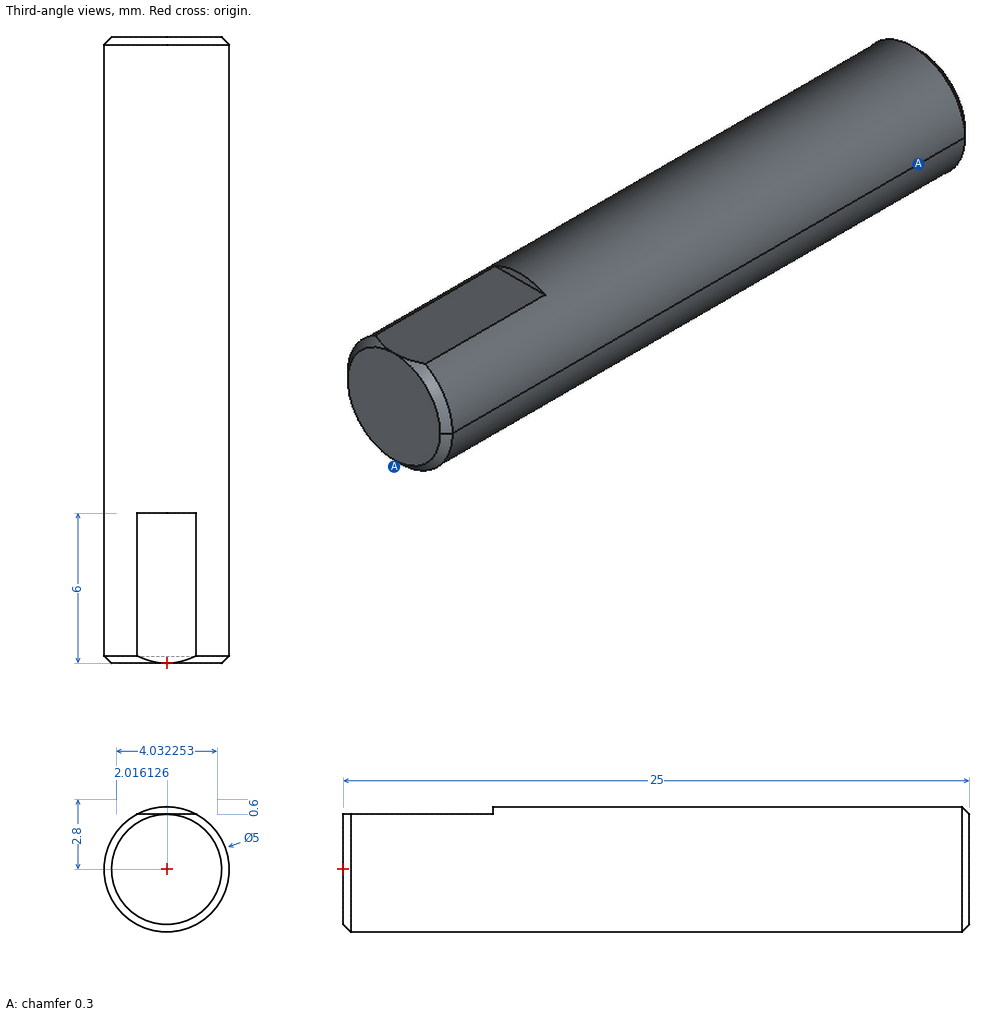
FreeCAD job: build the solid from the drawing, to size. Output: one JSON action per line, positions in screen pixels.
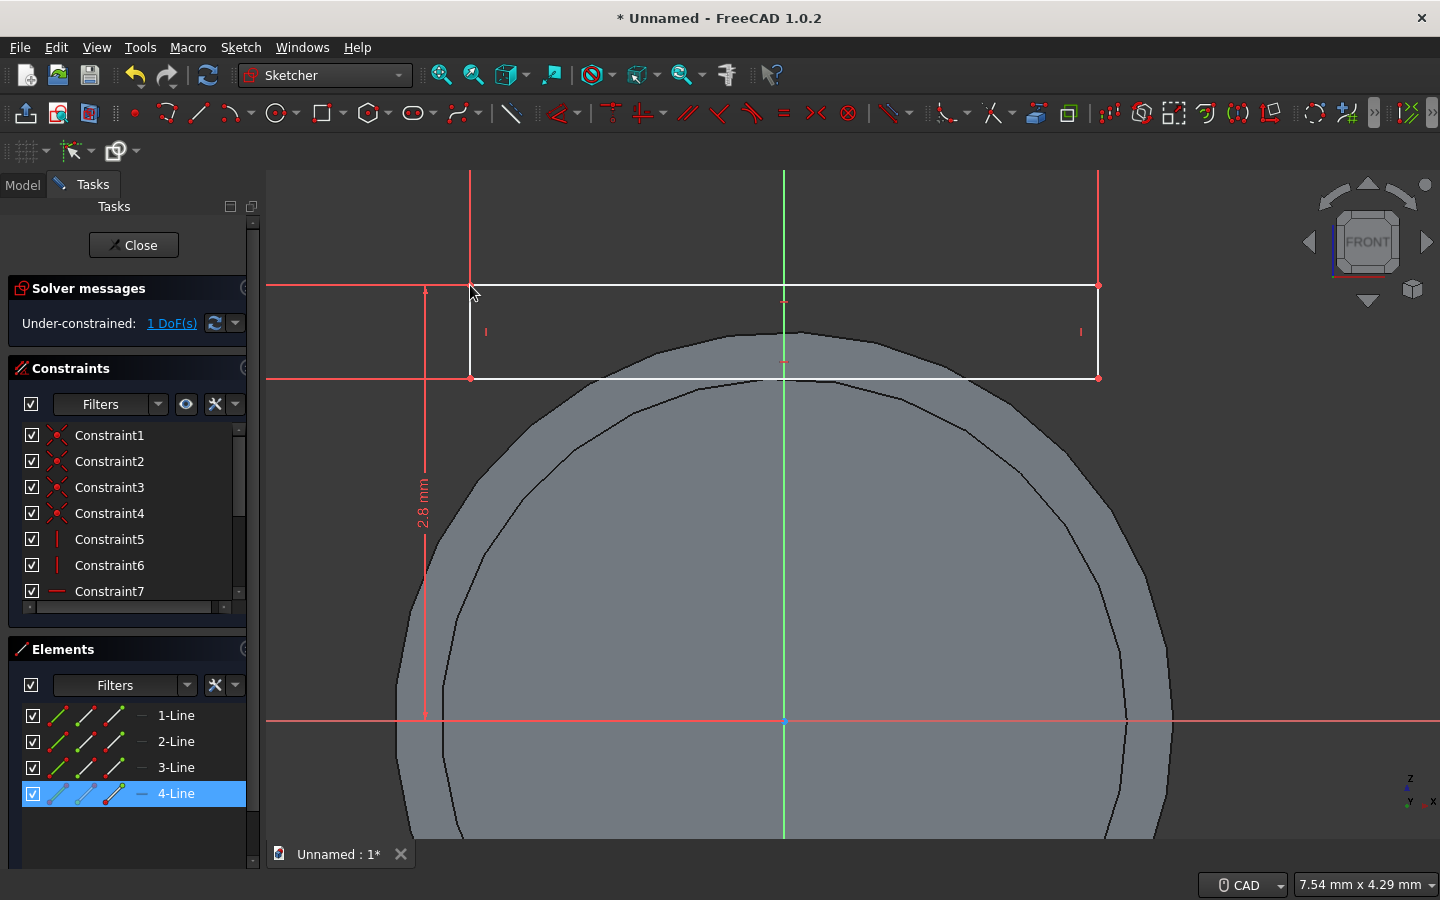
{"action": "key", "text": "l"}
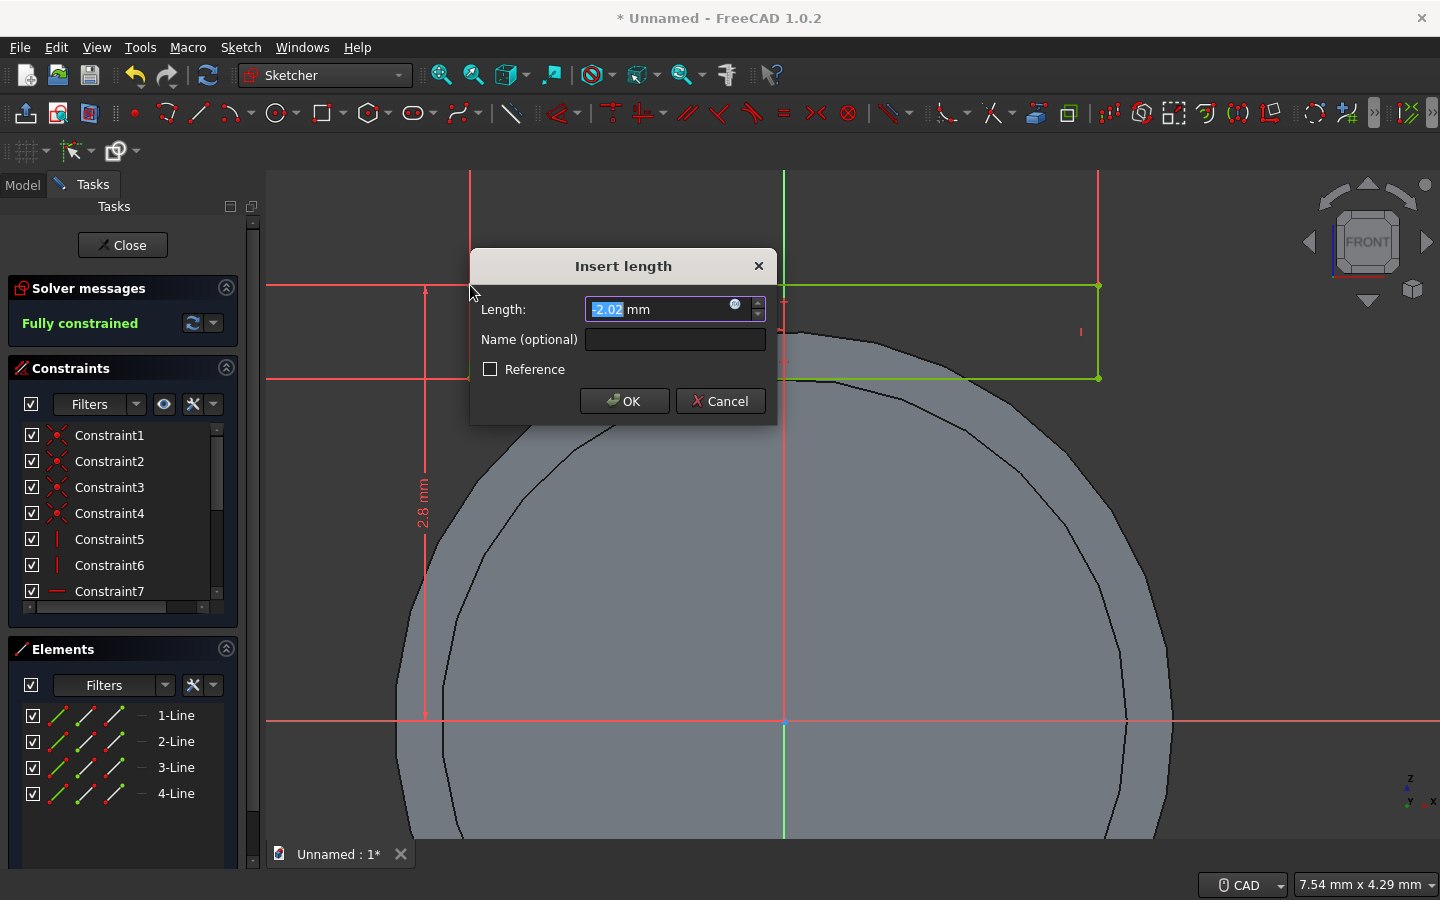
{"action": "type", "text": "-2.016126"}
{"action": "key", "text": "Return"}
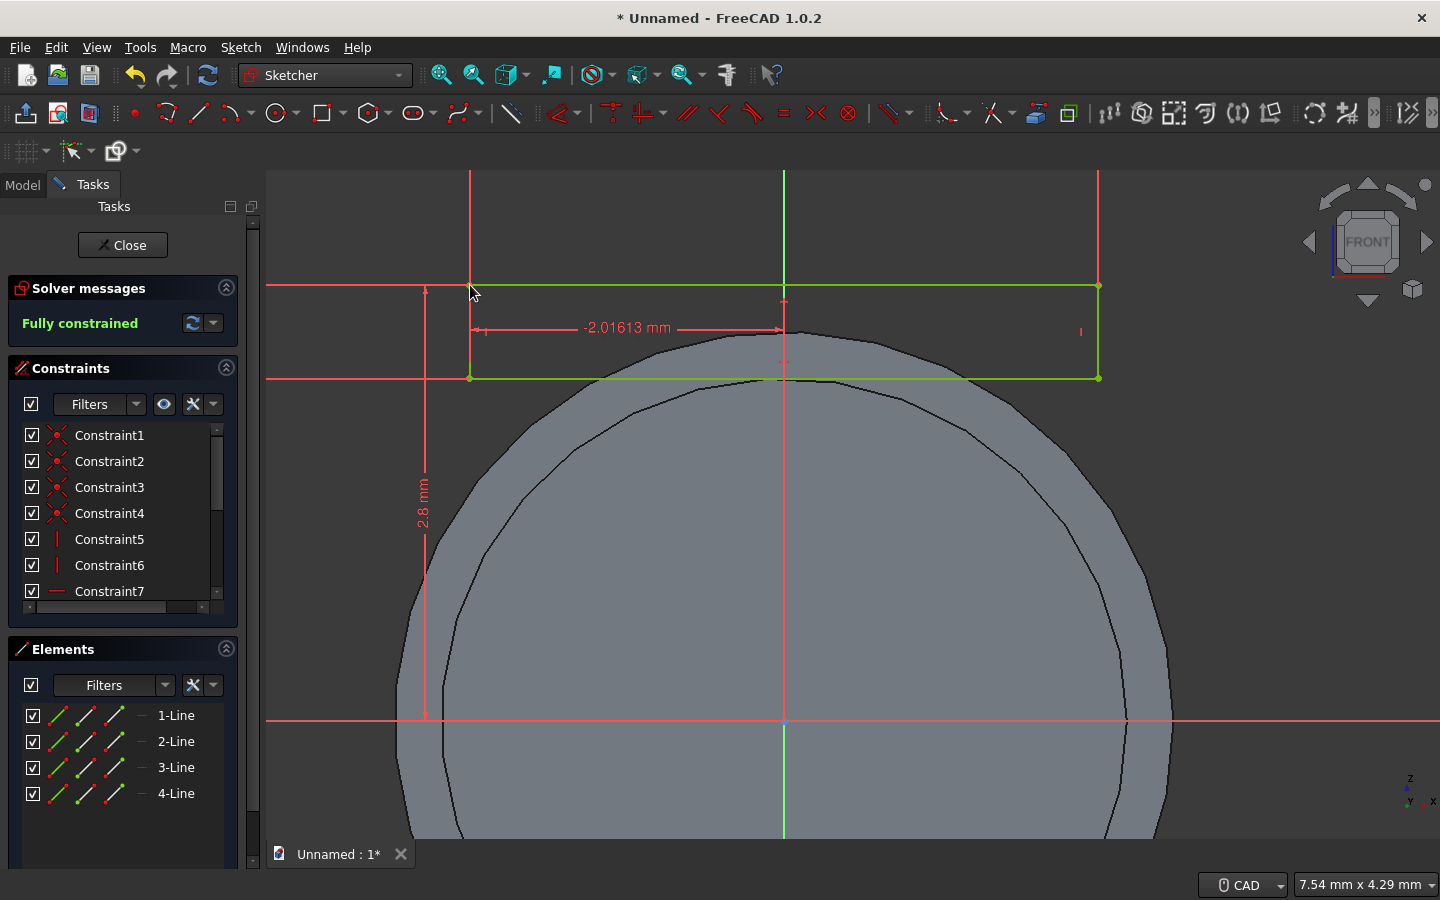
{"action": "left_click", "coordinate": [123, 245]}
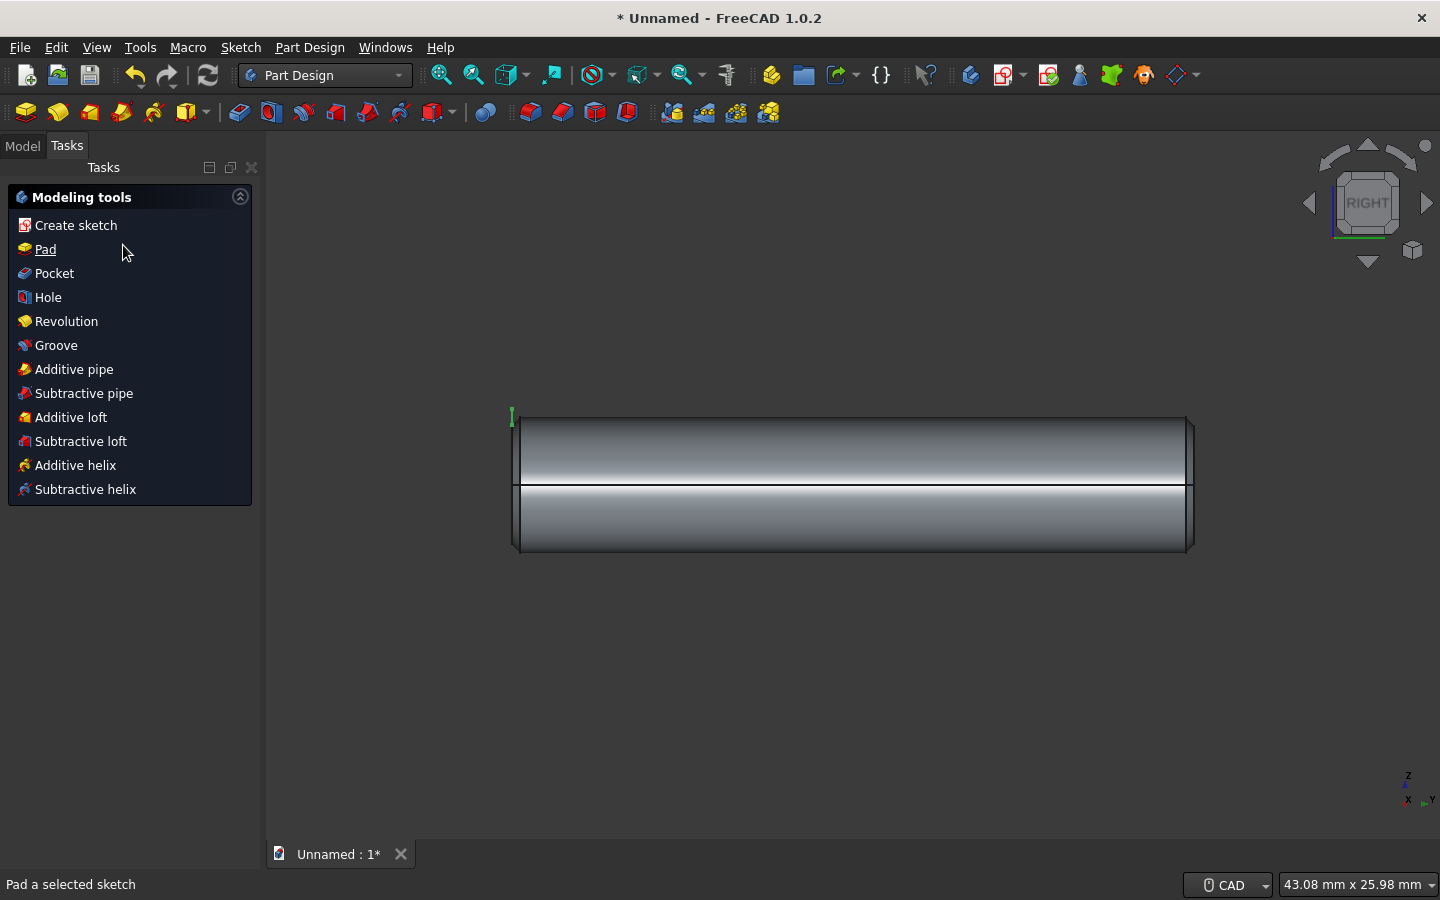
{"action": "left_click", "coordinate": [240, 112]}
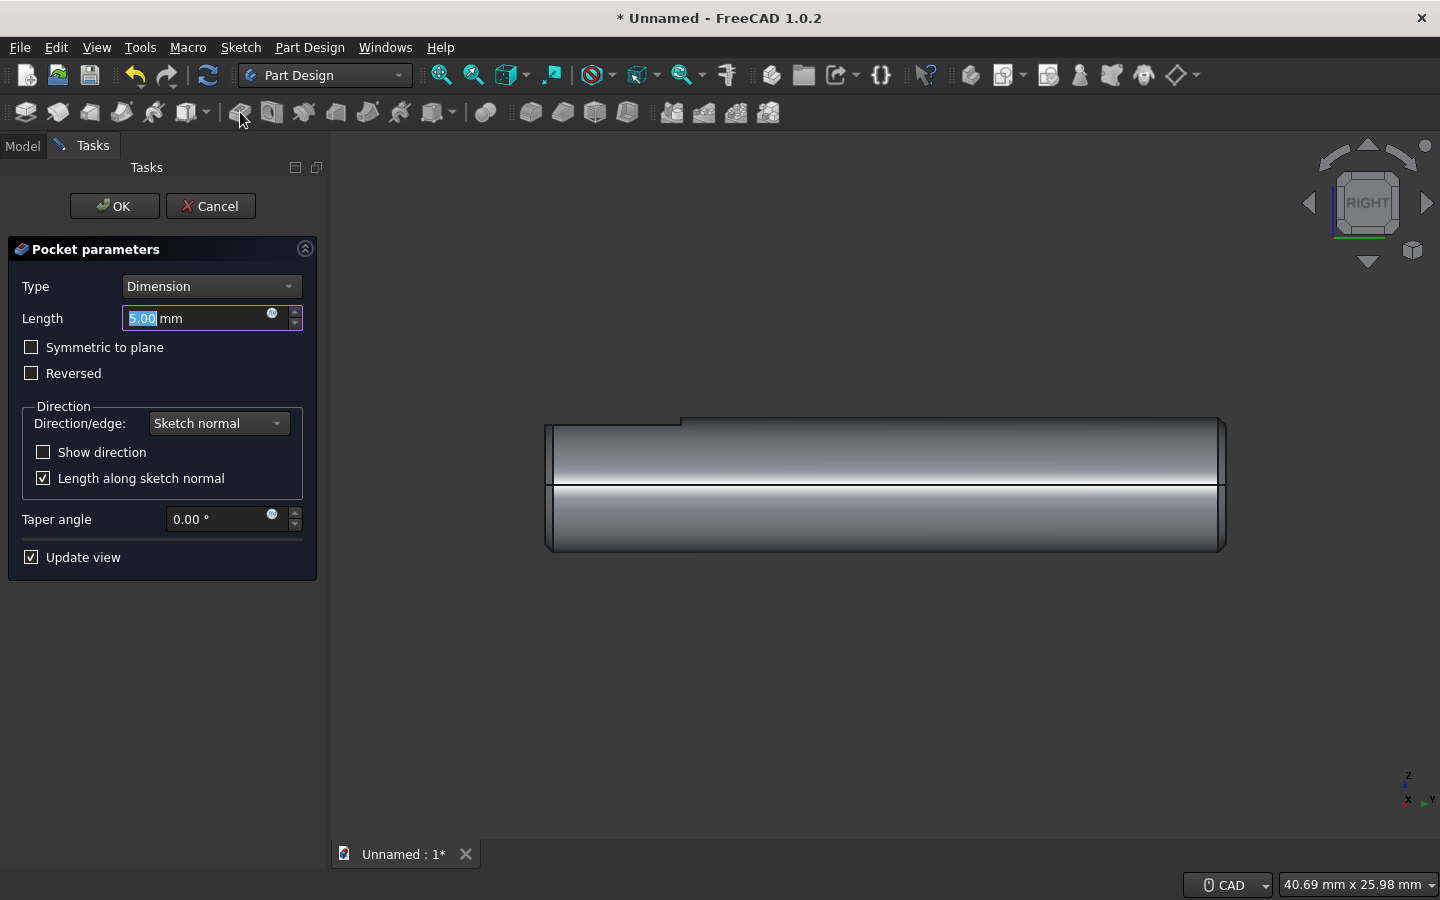
{"action": "type", "text": "6"}
{"action": "key", "text": "Tab"}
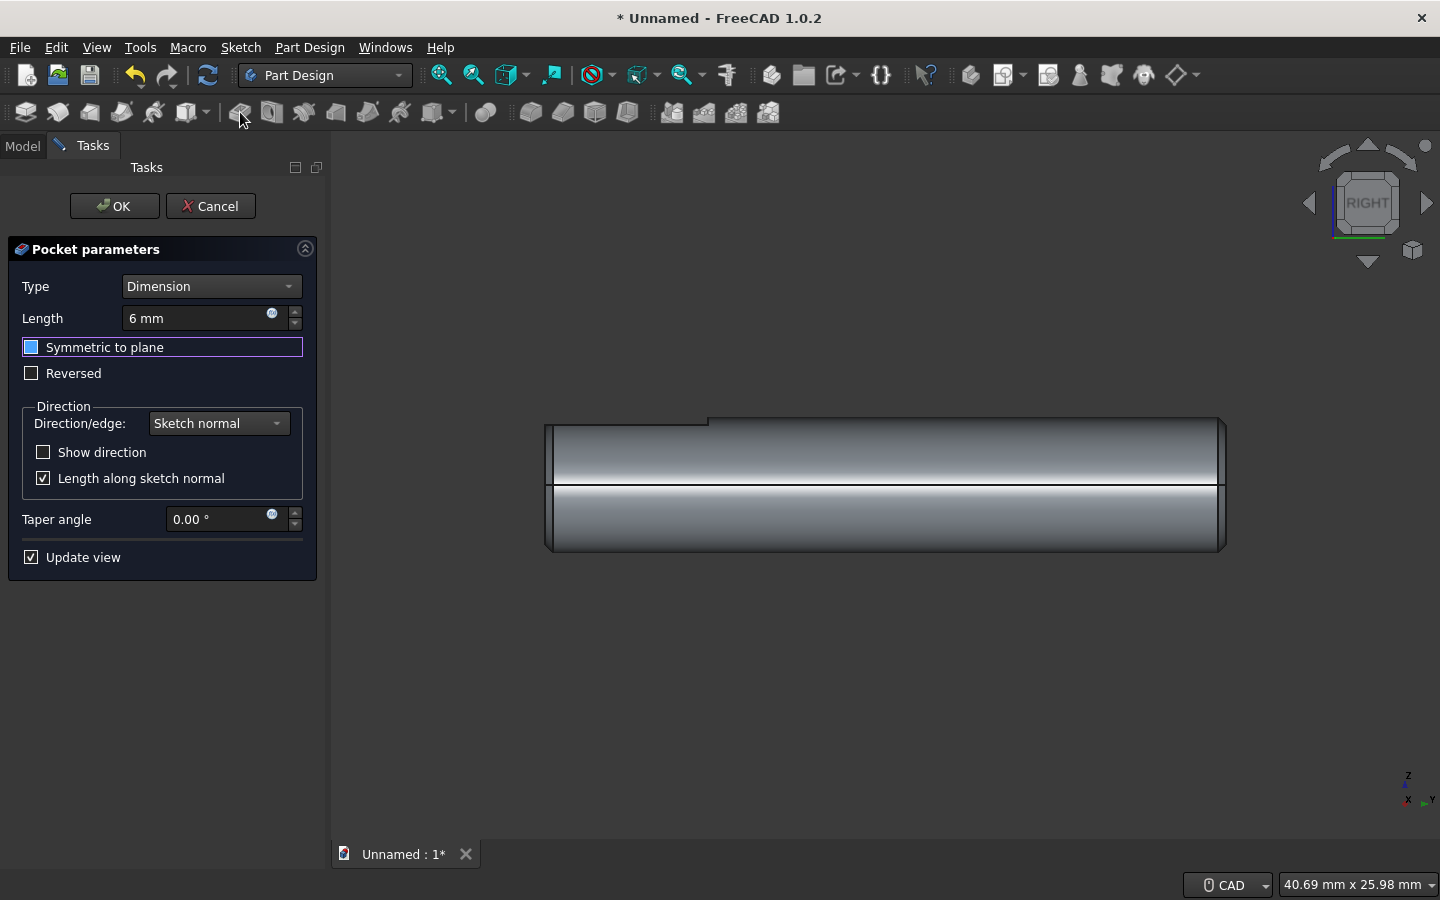
{"action": "left_click", "coordinate": [115, 206]}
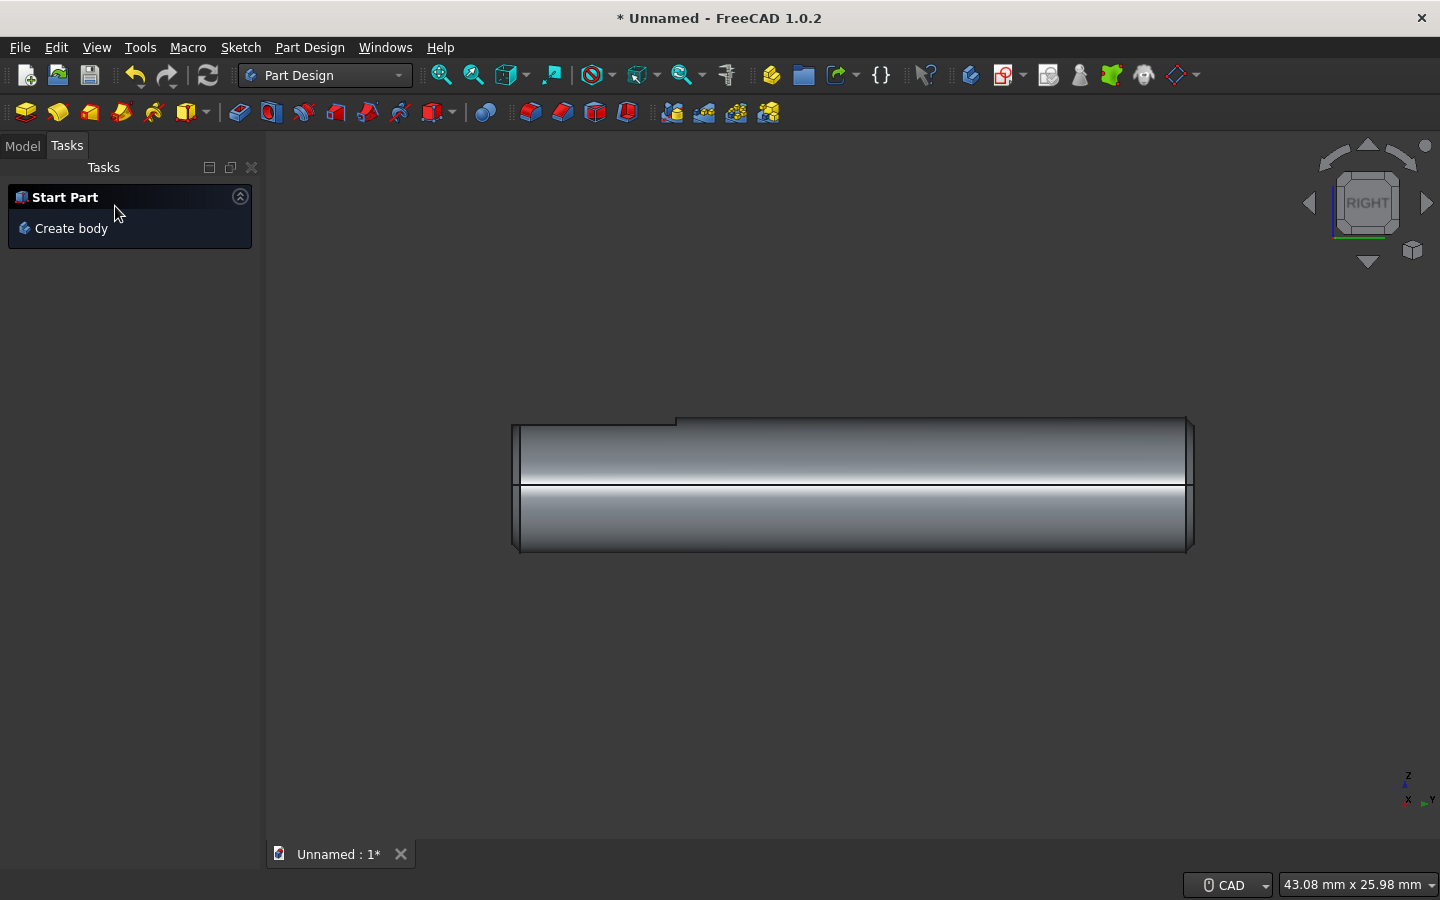
{"action": "key", "text": "0"}